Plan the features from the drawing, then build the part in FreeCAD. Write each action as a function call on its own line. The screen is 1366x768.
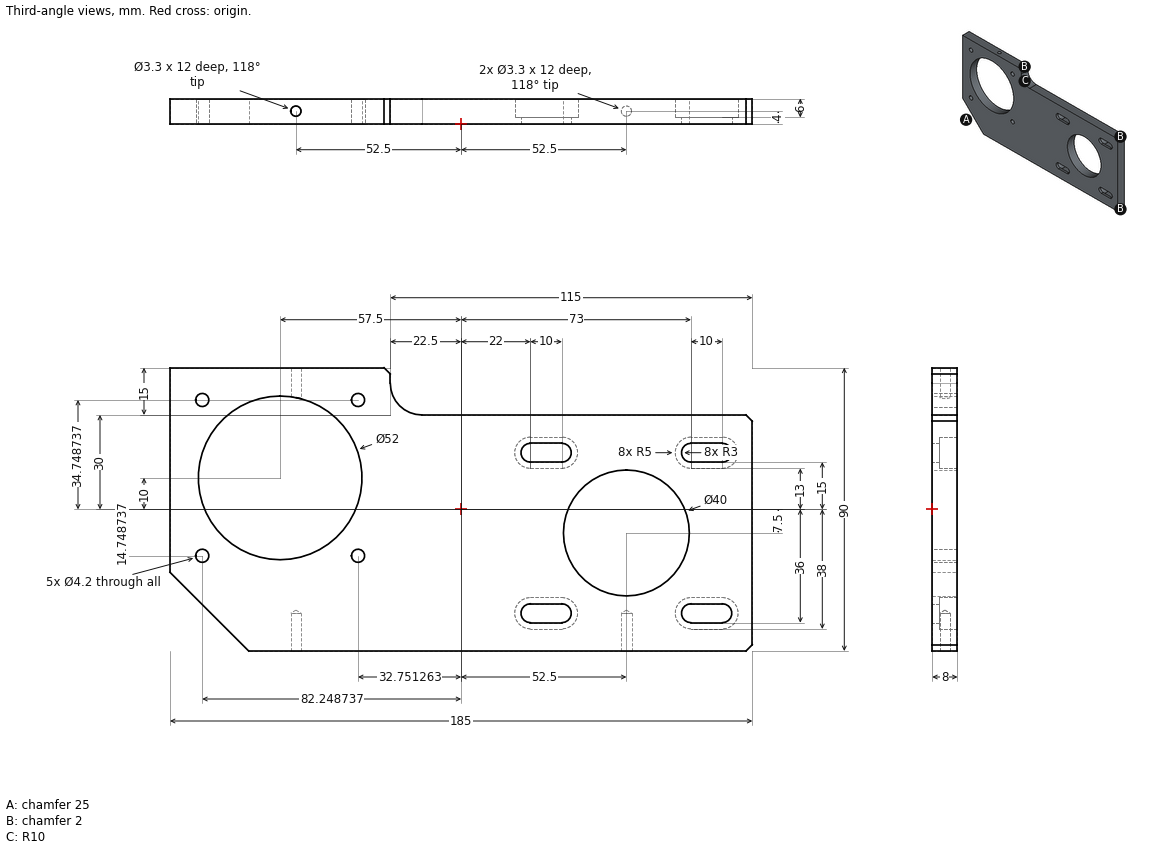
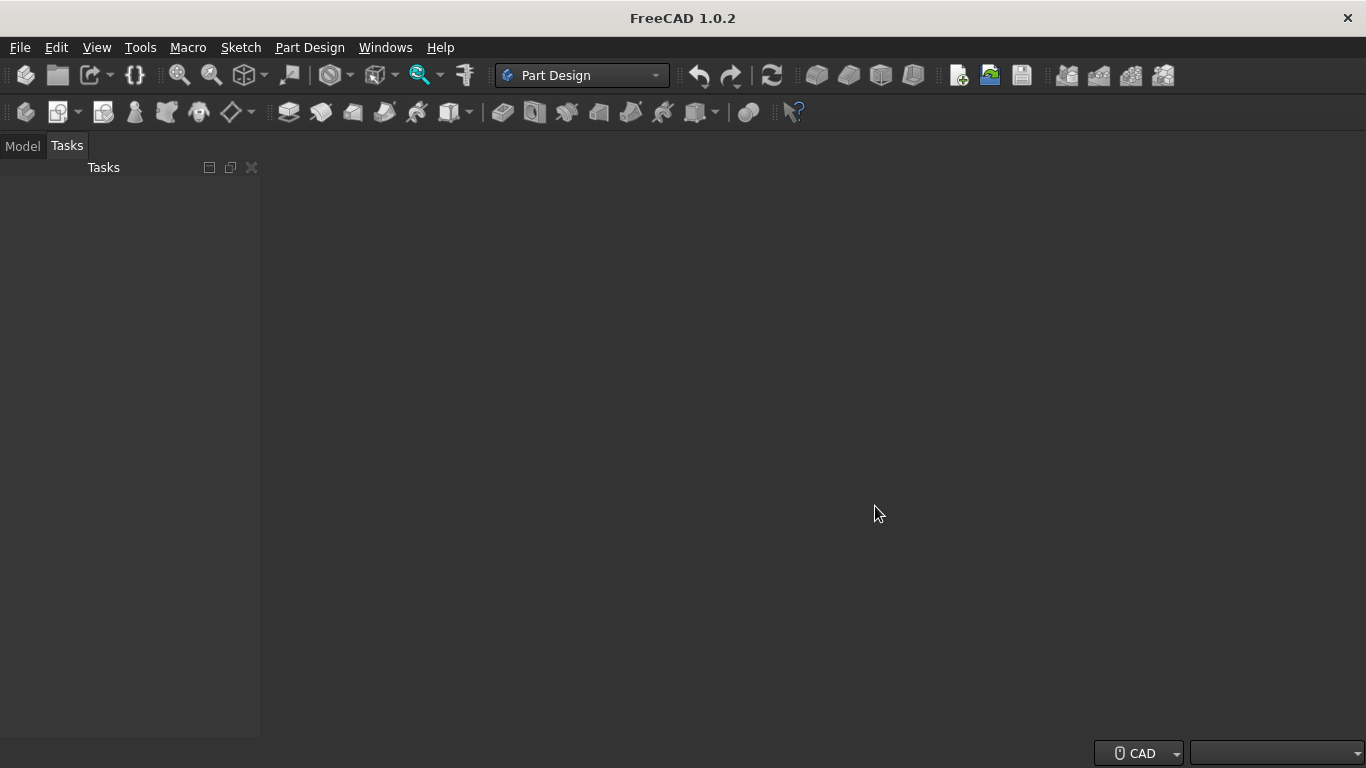
click(958, 76)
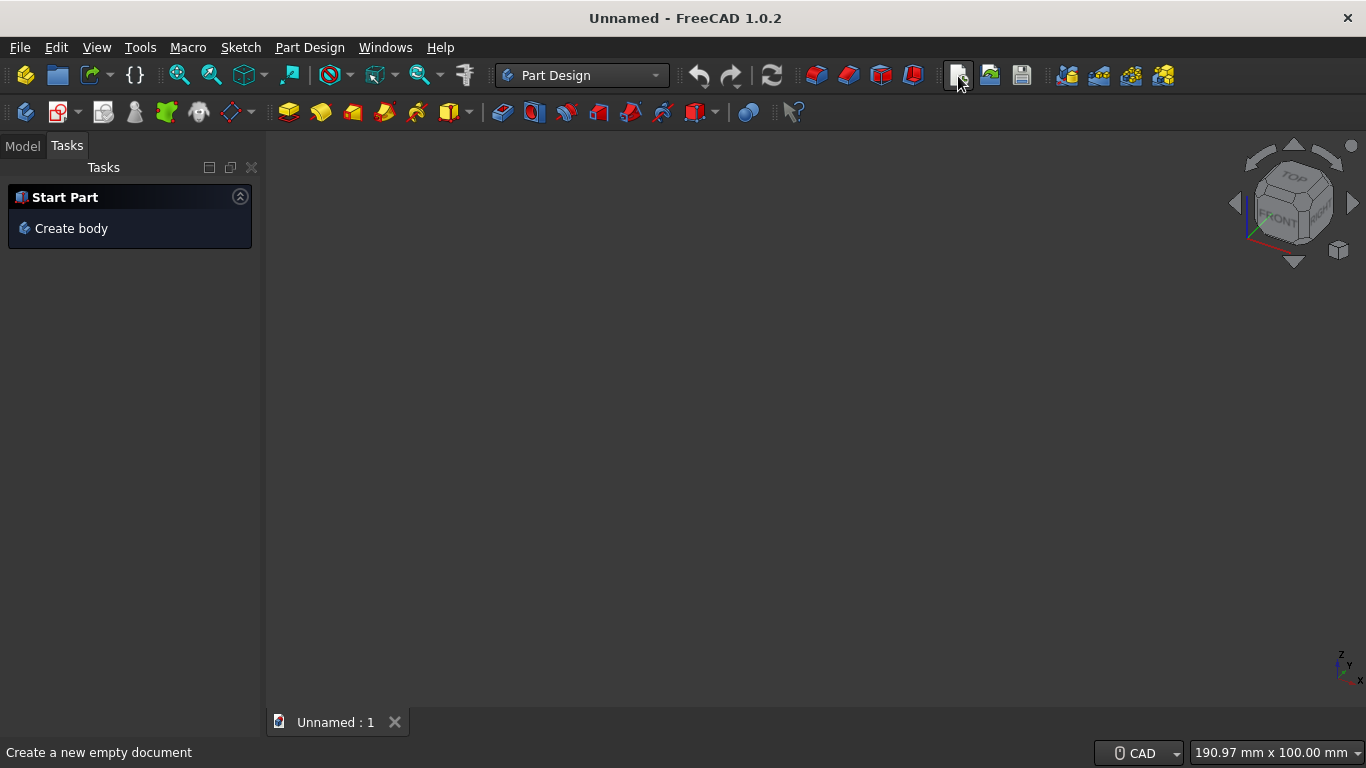
click(58, 112)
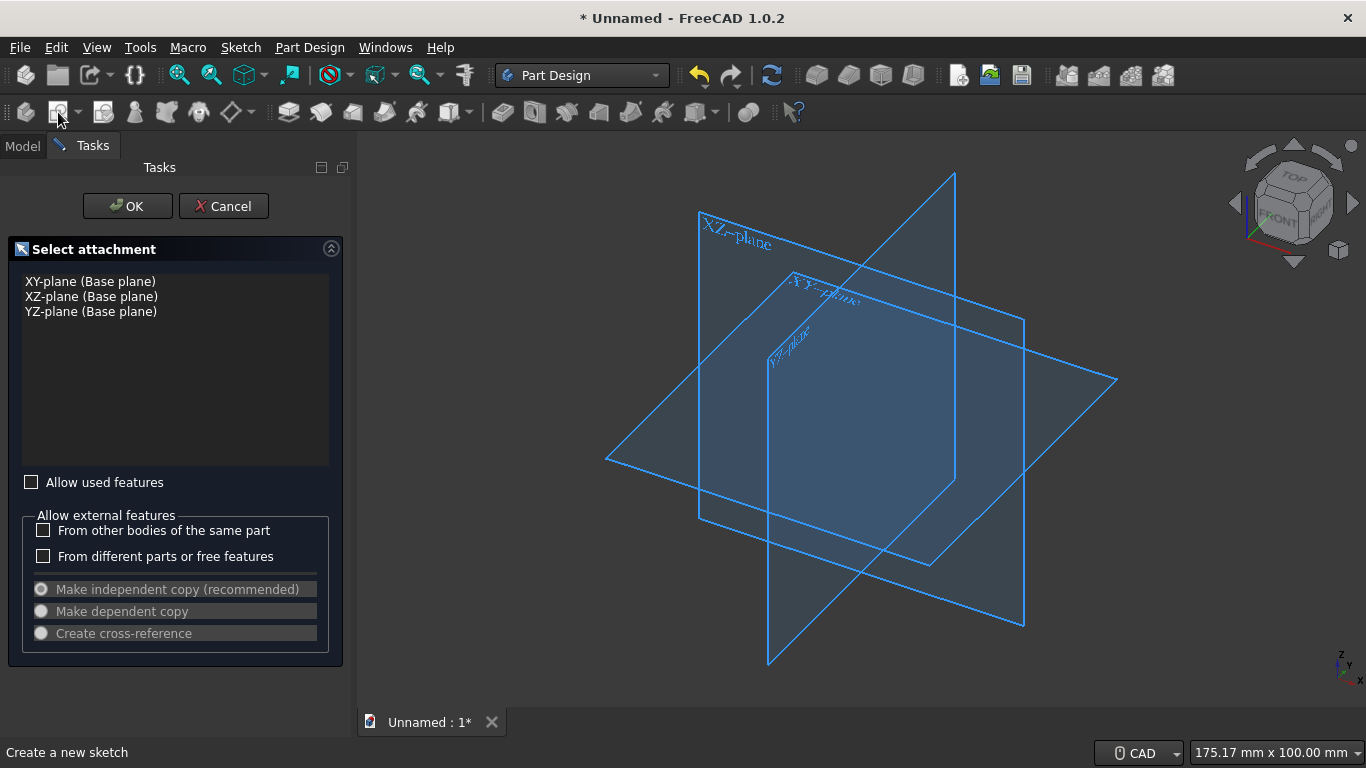
click(82, 296)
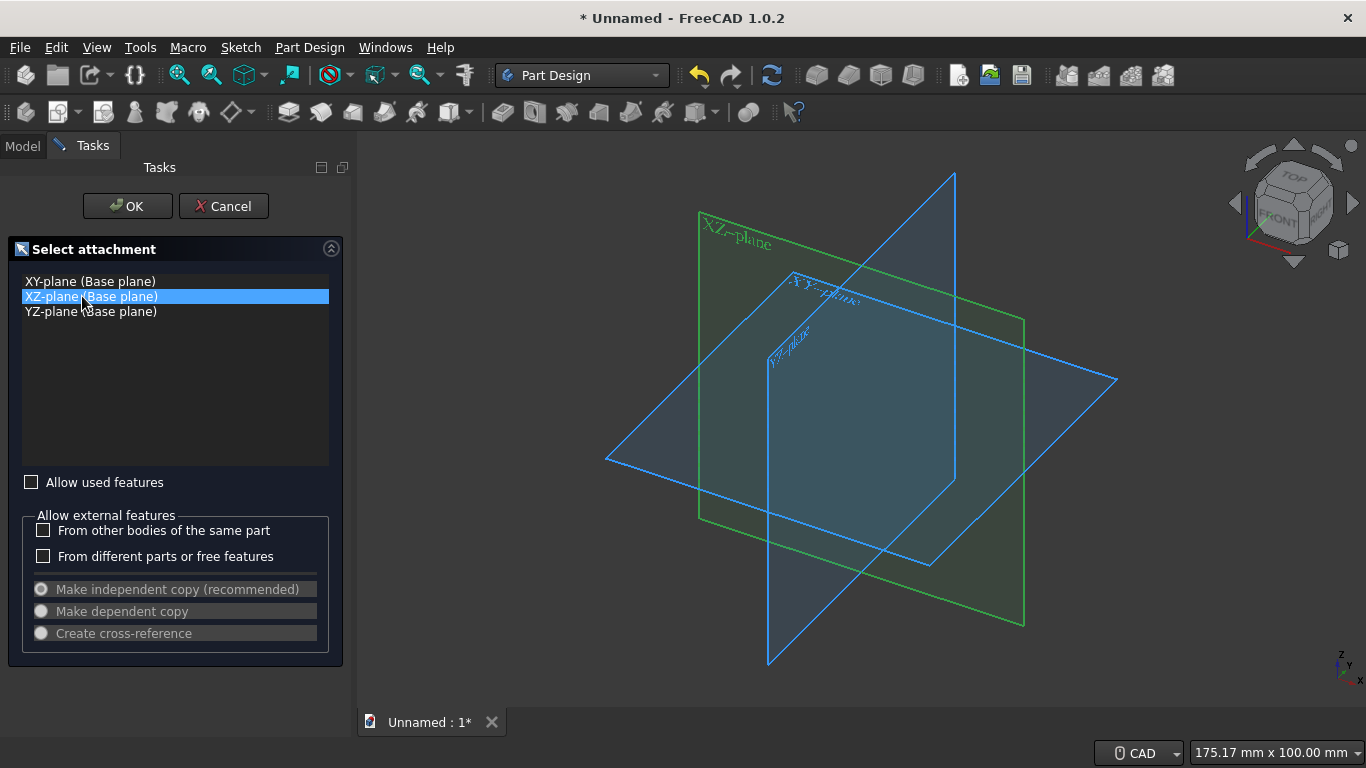
click(128, 206)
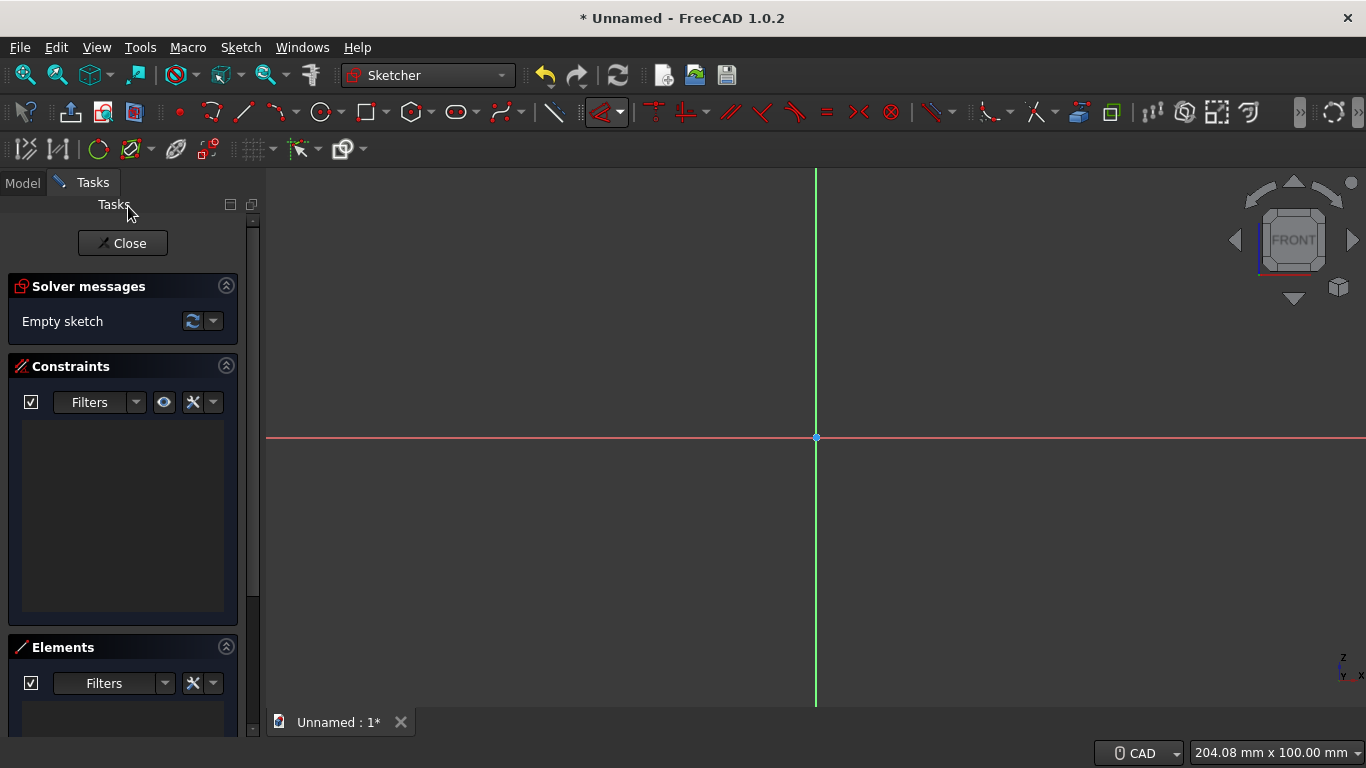
scroll(608, 438, down, 2)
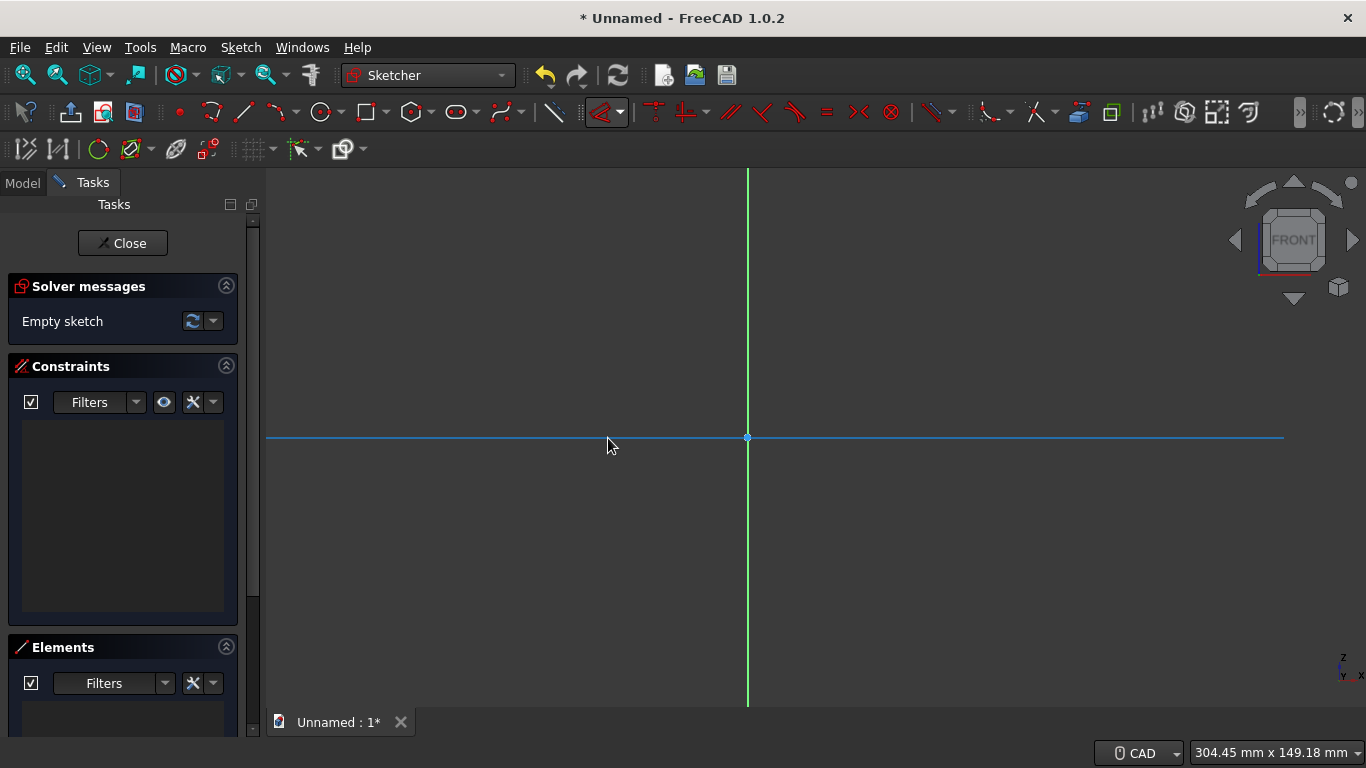
click(388, 112)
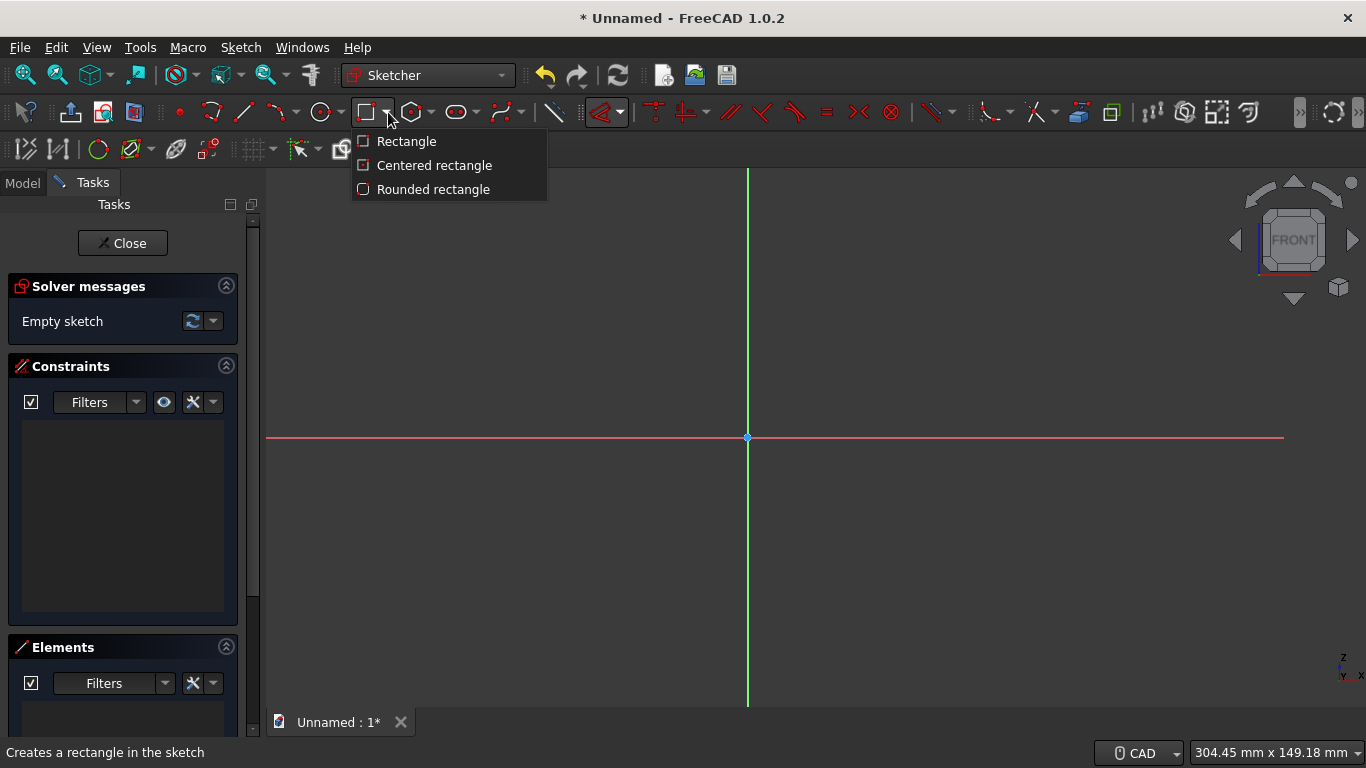
click(450, 165)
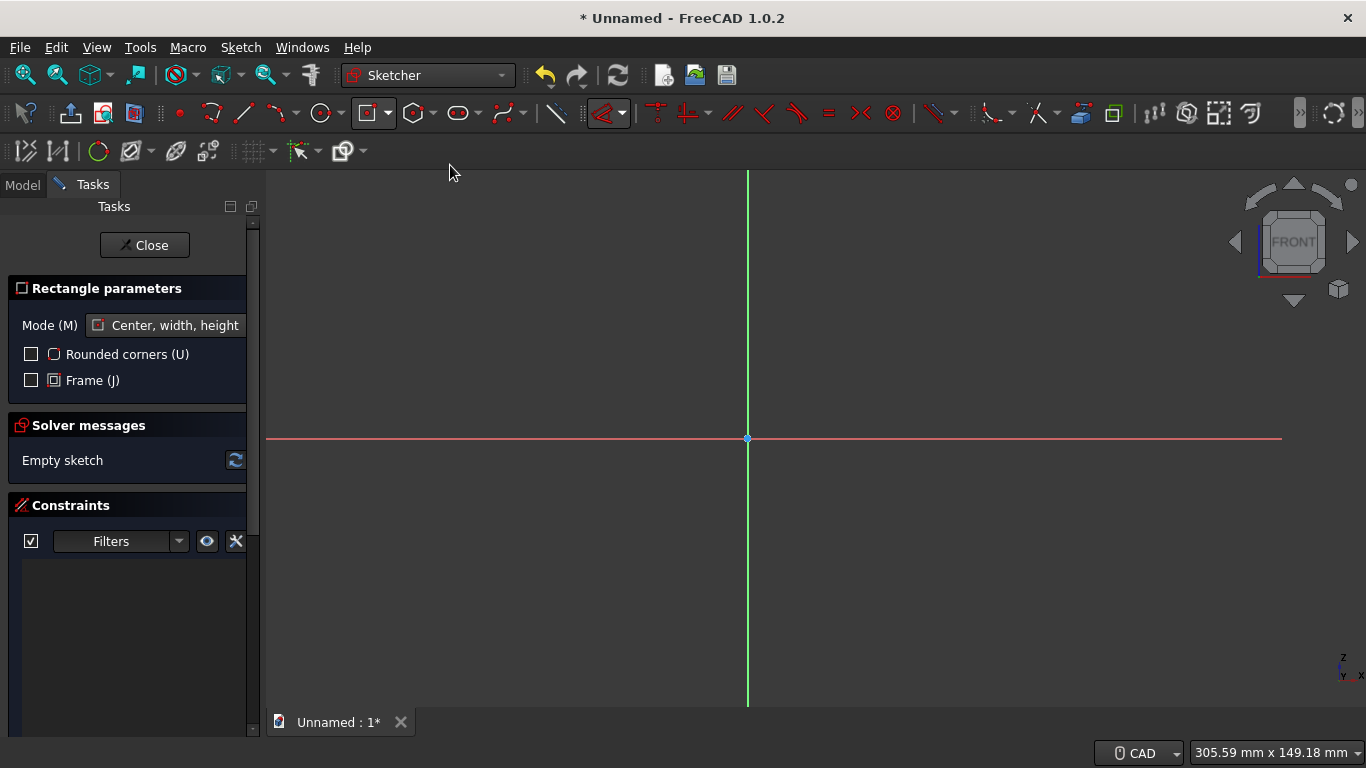
click(748, 439)
click(1081, 277)
key(Escape)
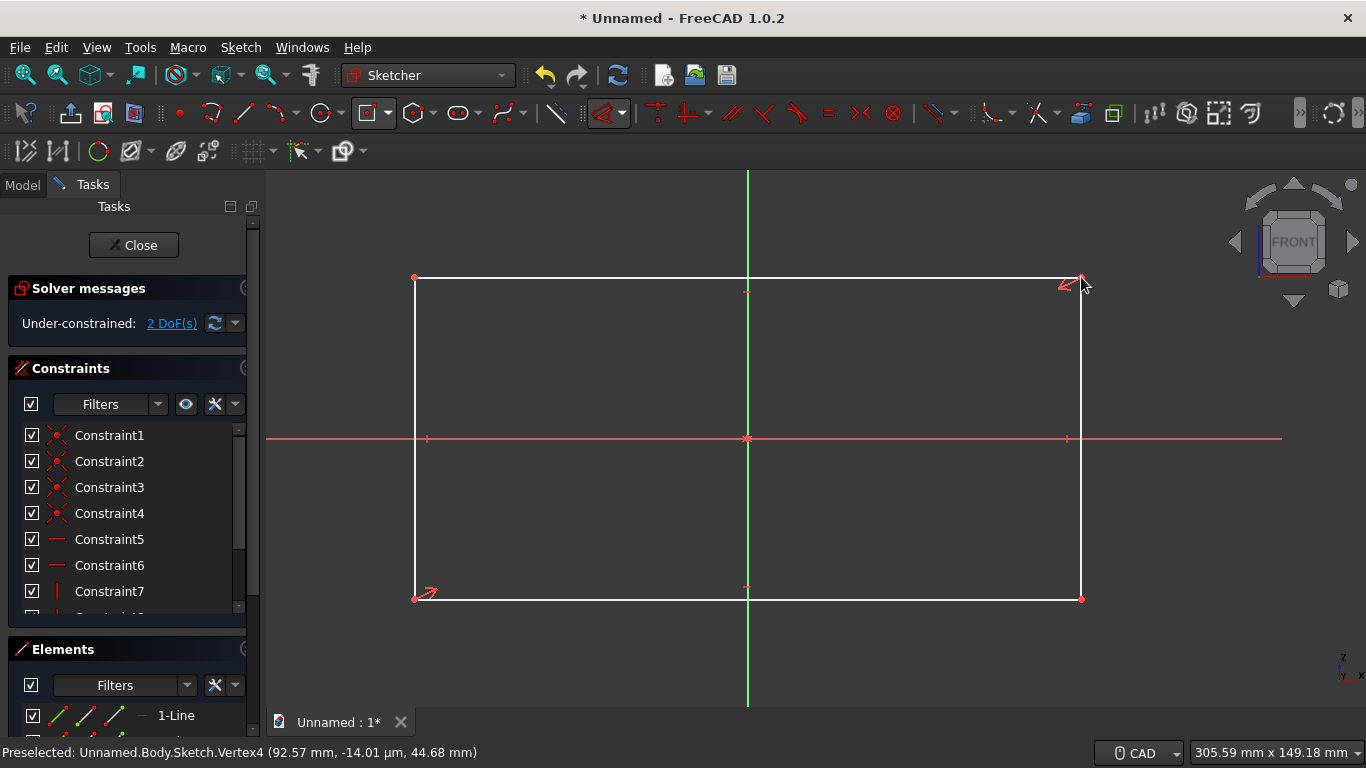
click(1081, 503)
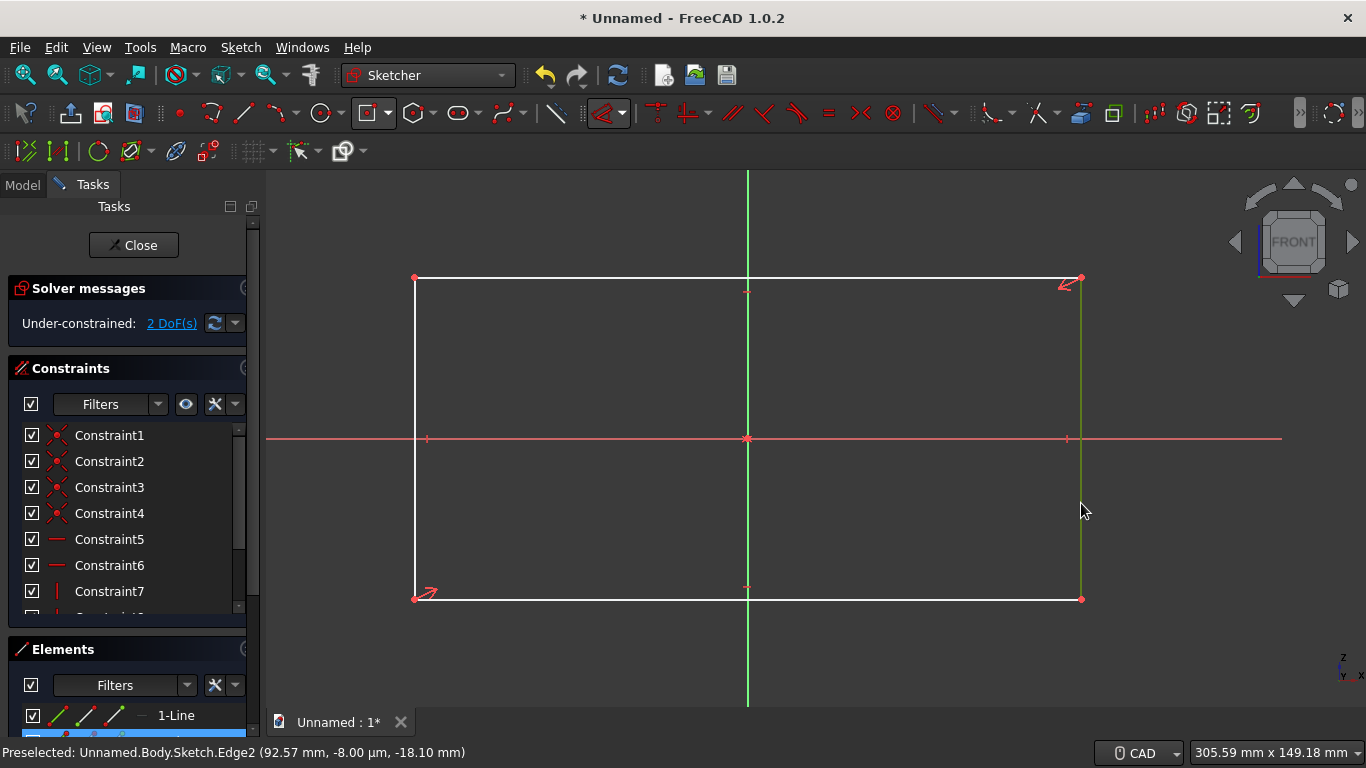
click(624, 114)